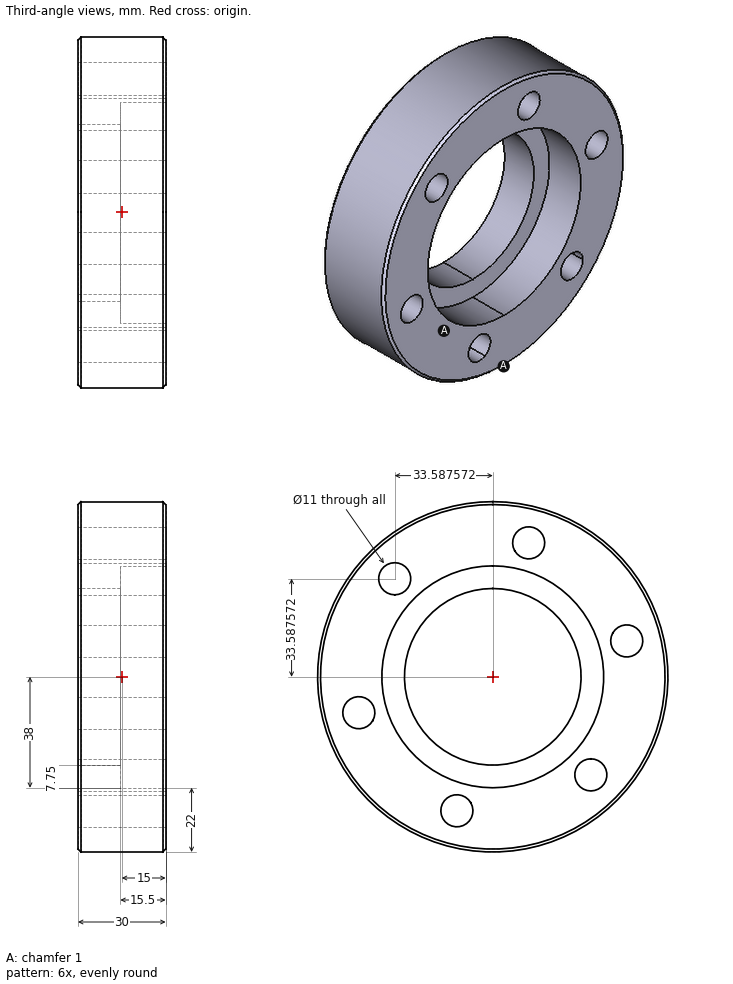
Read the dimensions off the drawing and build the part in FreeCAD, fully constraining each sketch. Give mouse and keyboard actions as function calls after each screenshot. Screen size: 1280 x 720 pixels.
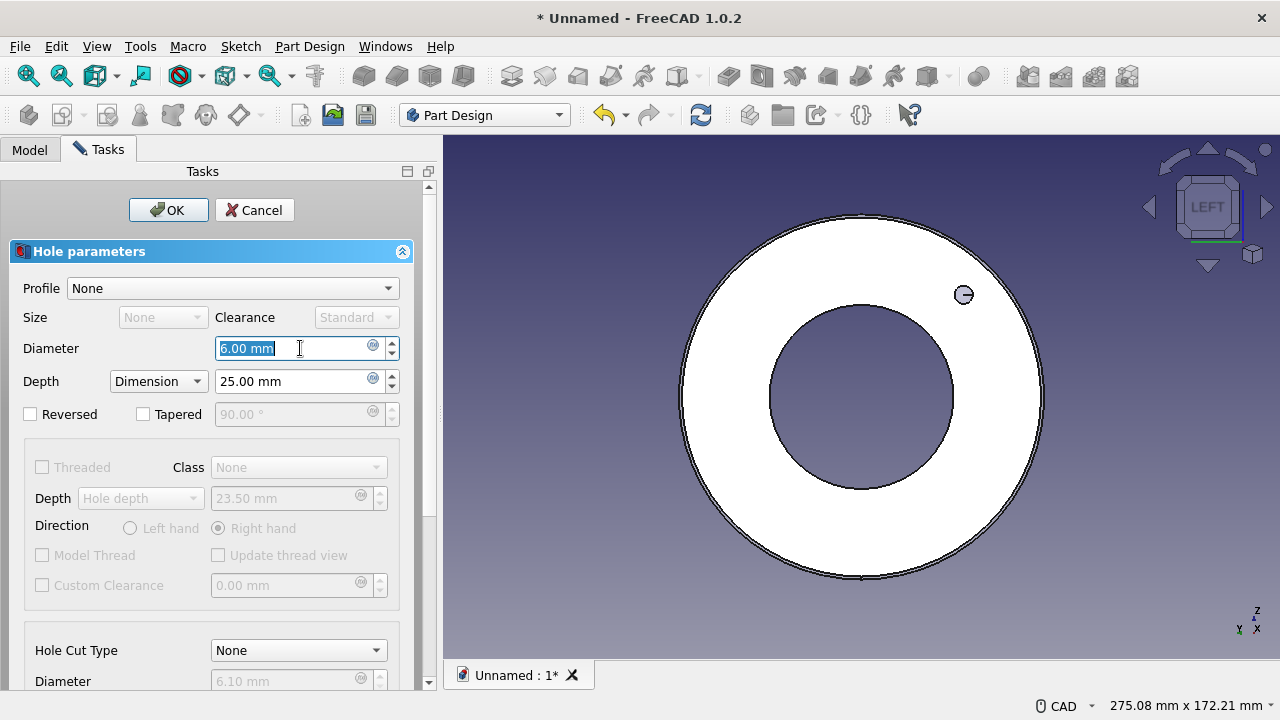
text(11)
key(Tab)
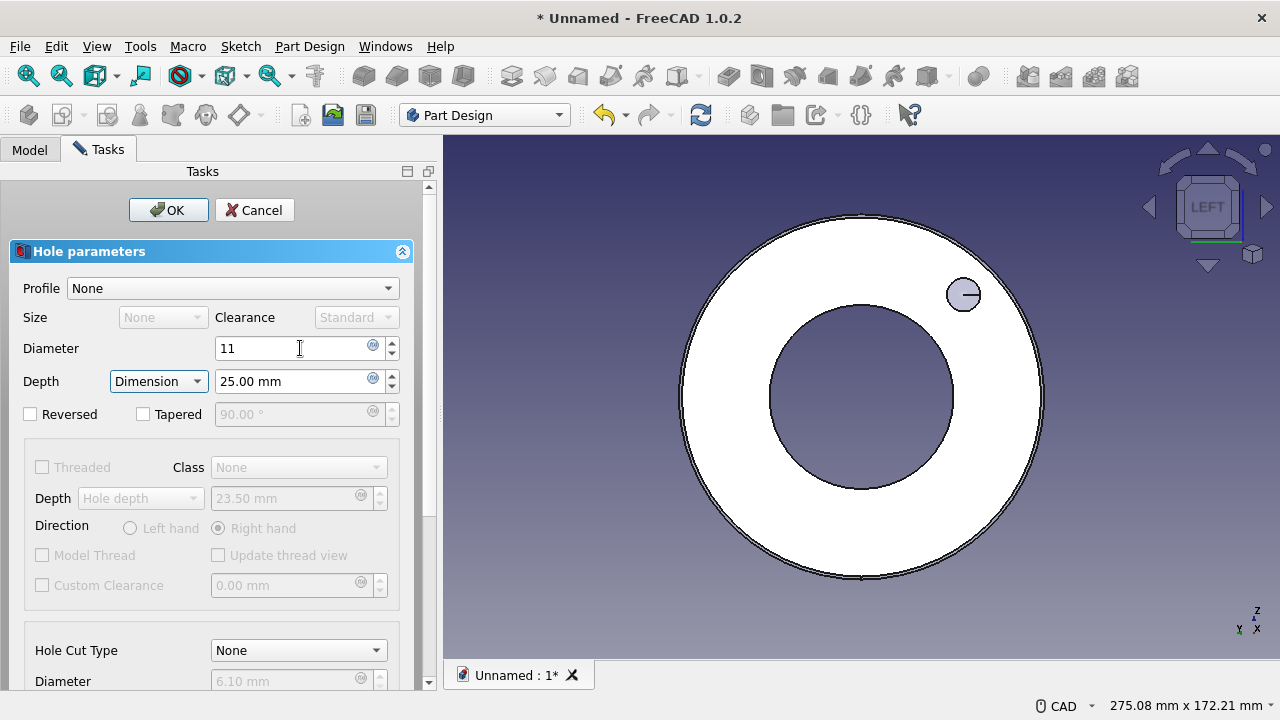
click(160, 382)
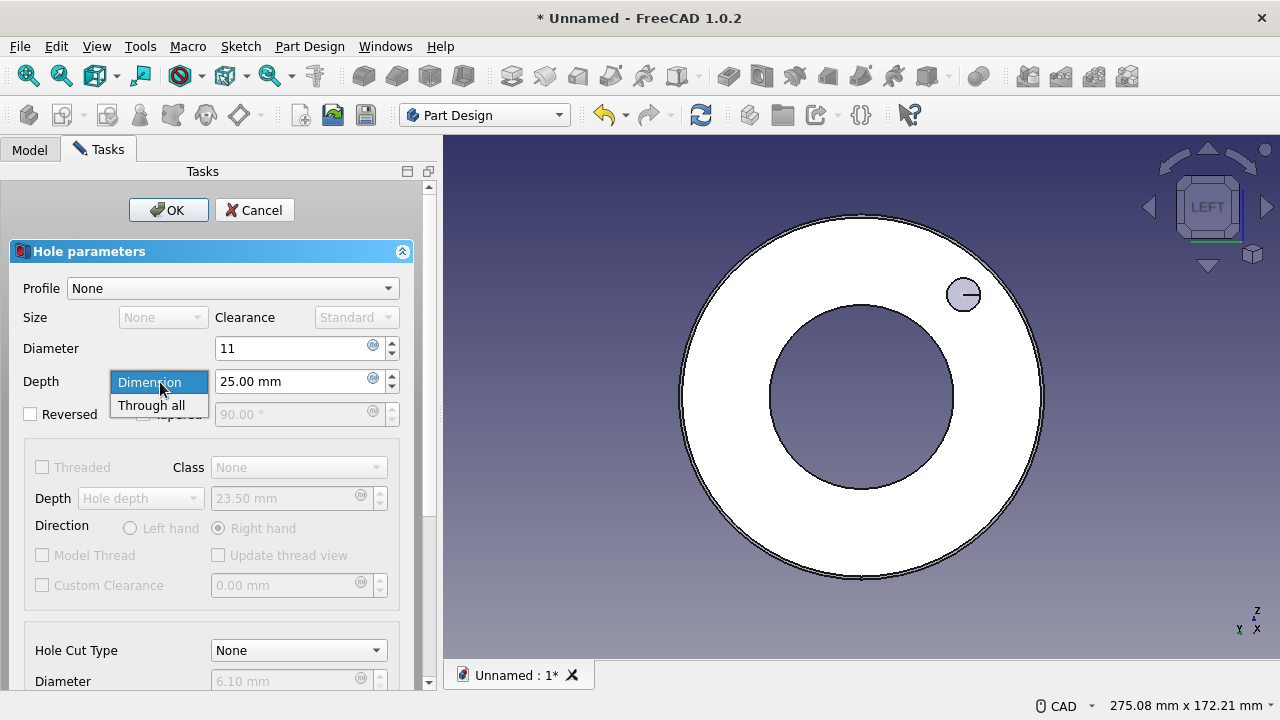
click(158, 406)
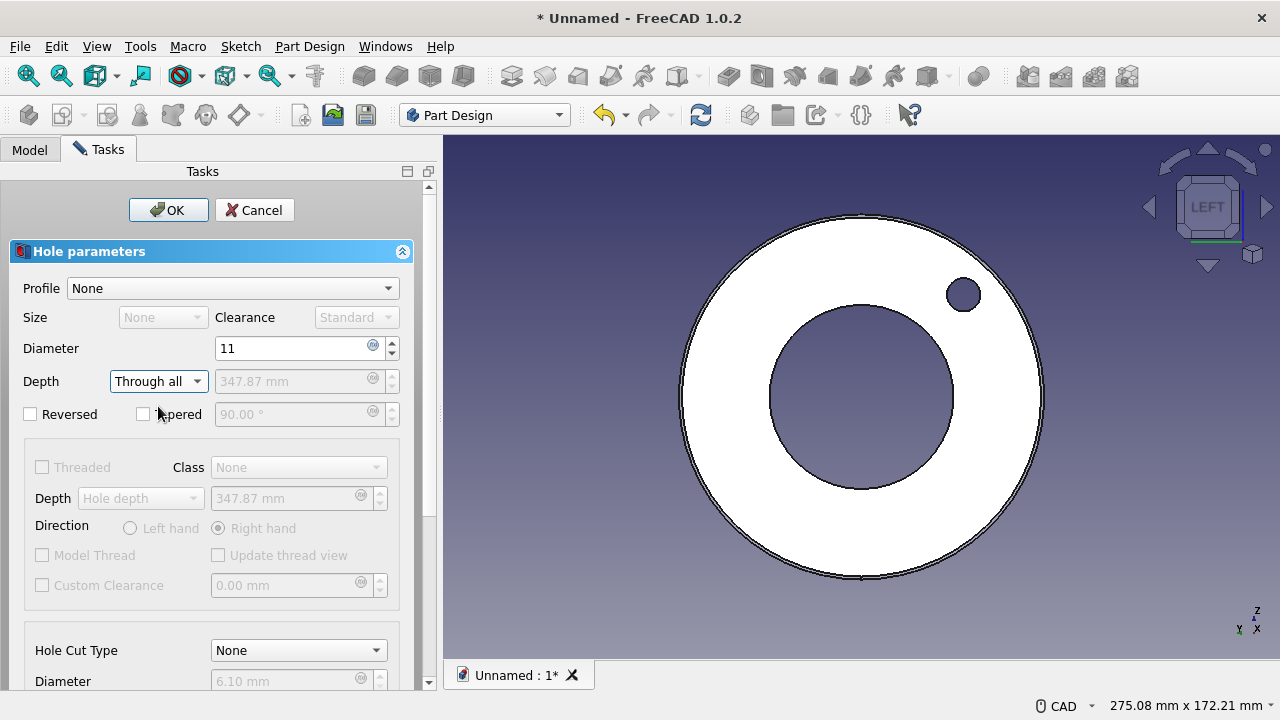
click(169, 210)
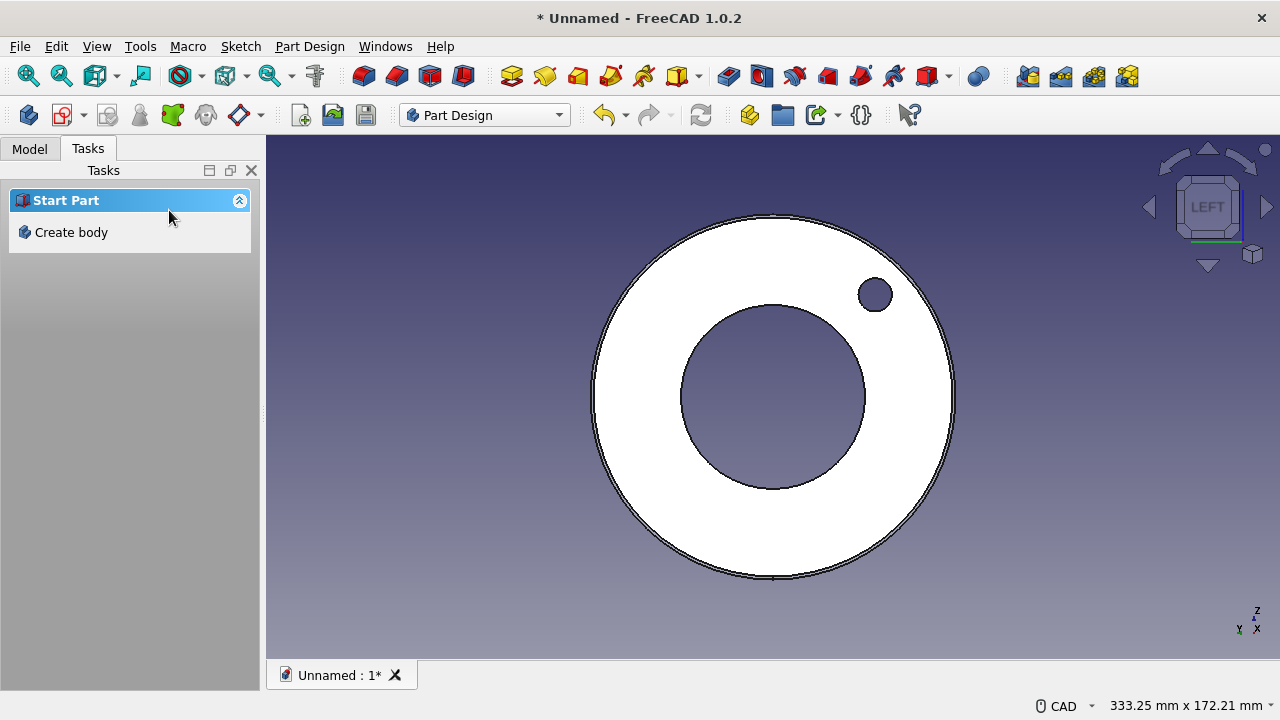
click(30, 148)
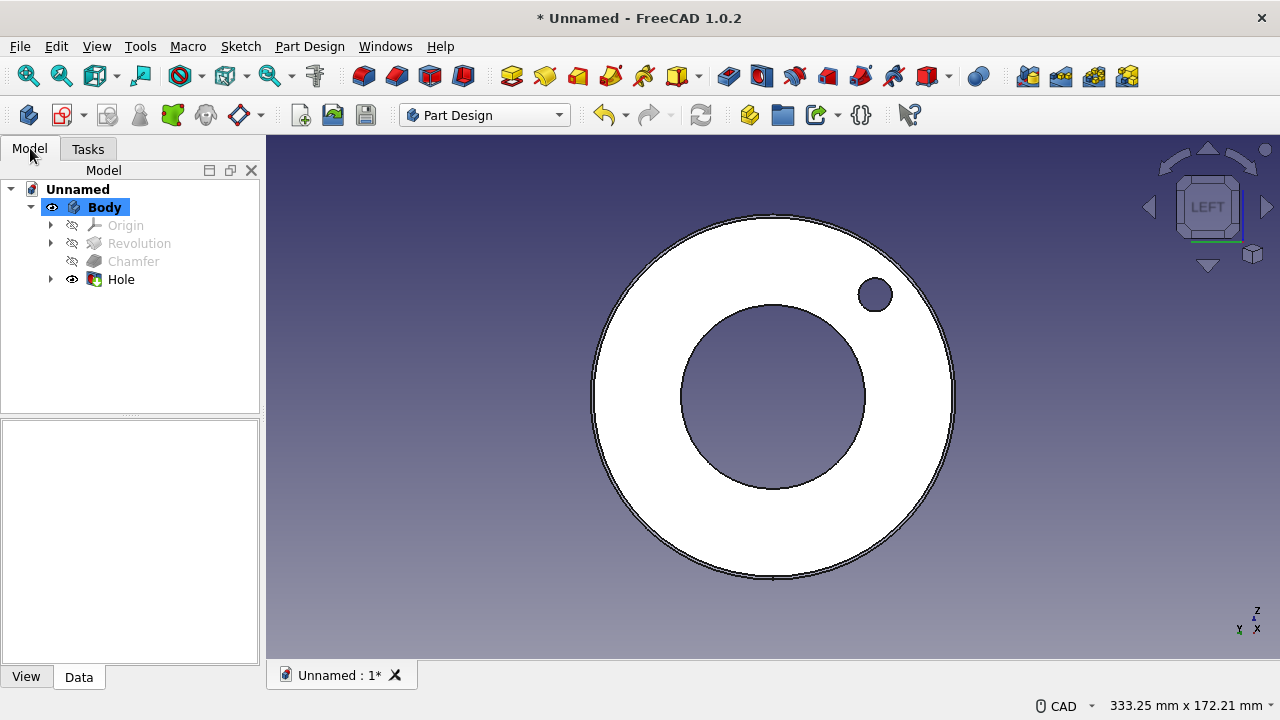
click(117, 279)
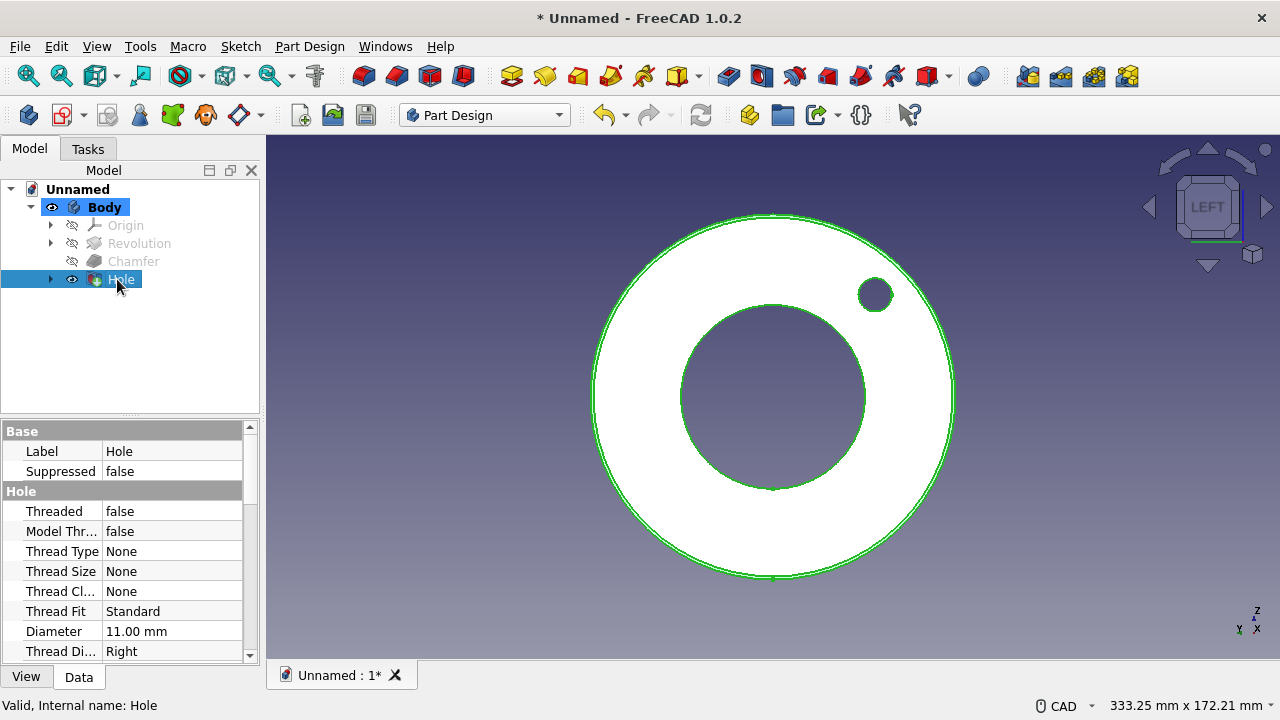
click(1094, 76)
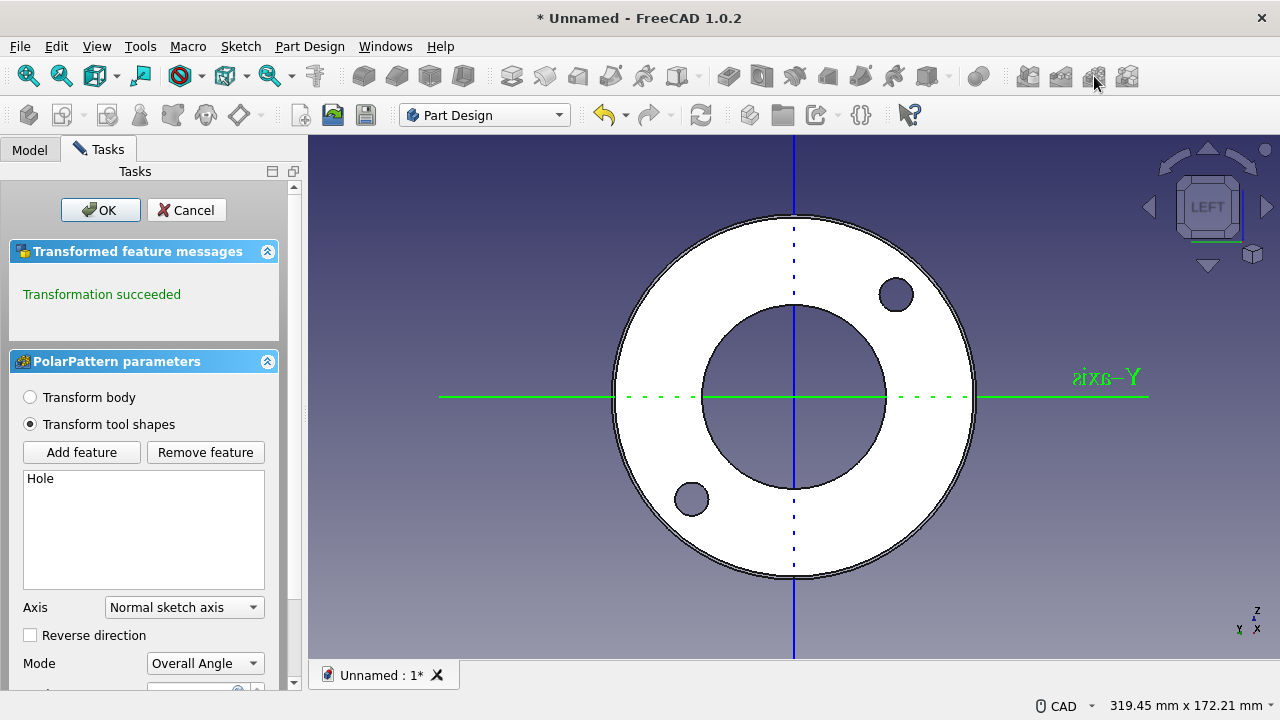
click(185, 608)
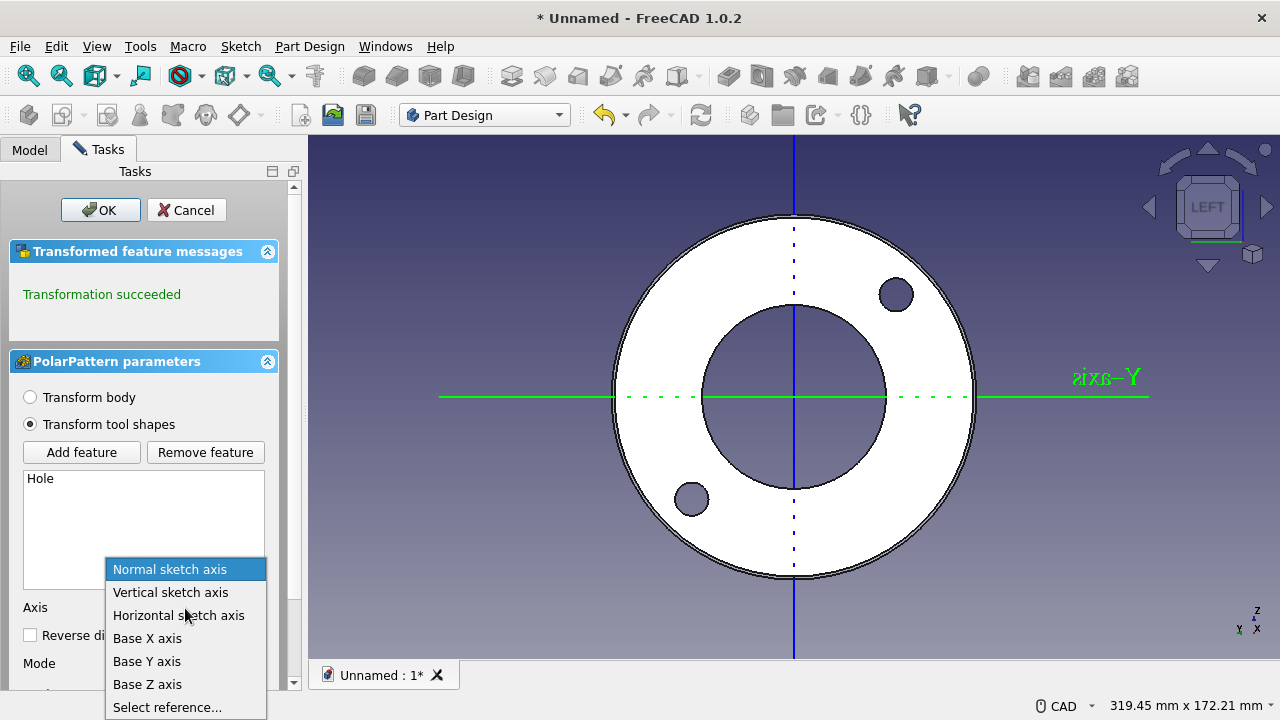
click(184, 638)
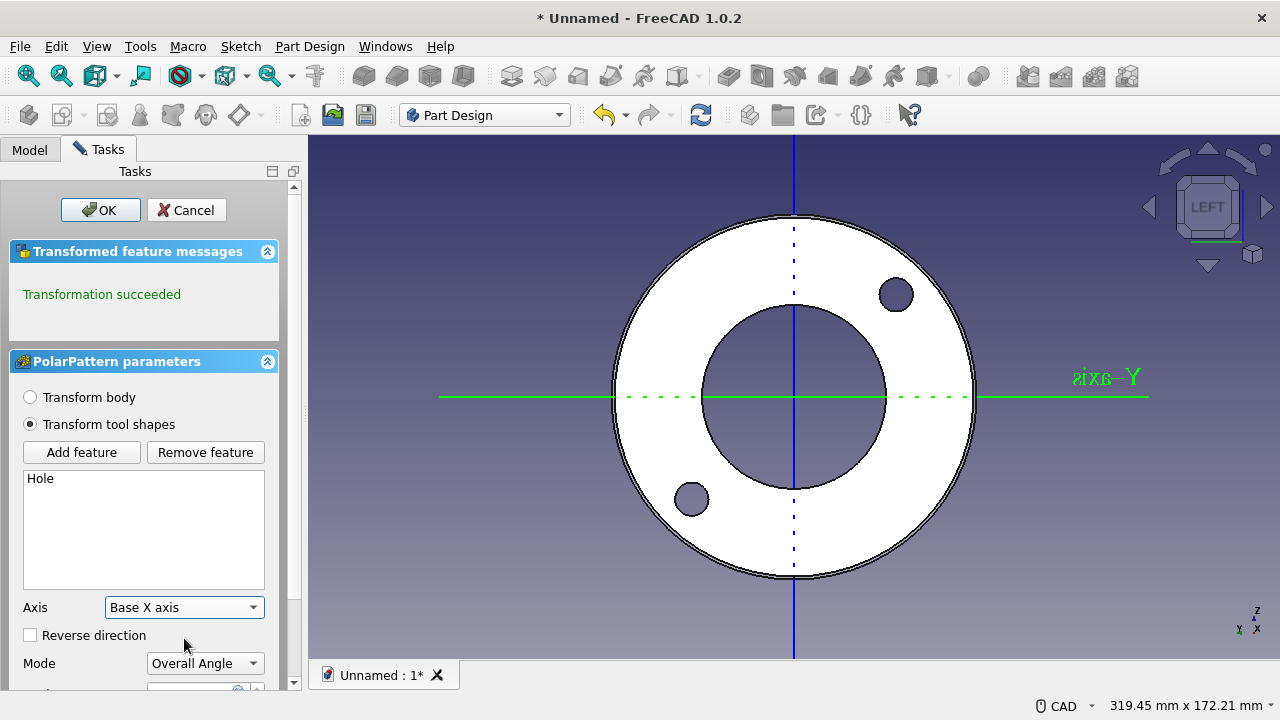
scroll(294, 436, down, 2)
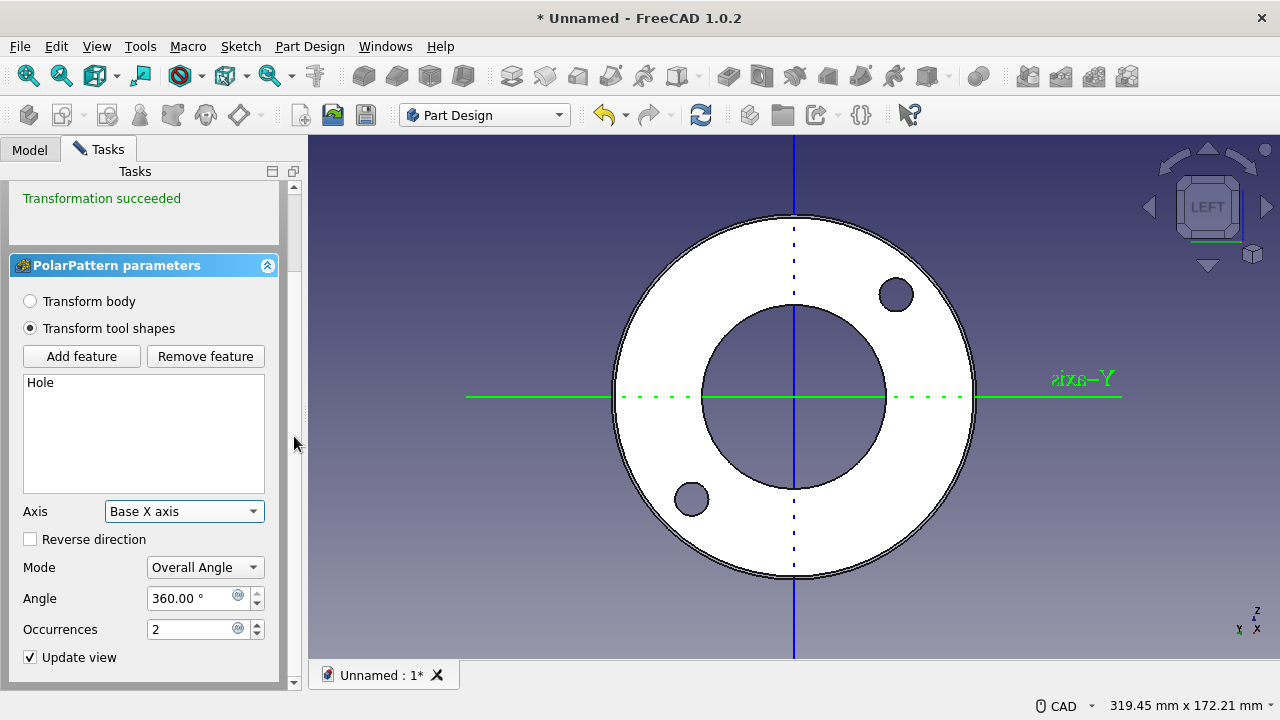
triple_click(199, 630)